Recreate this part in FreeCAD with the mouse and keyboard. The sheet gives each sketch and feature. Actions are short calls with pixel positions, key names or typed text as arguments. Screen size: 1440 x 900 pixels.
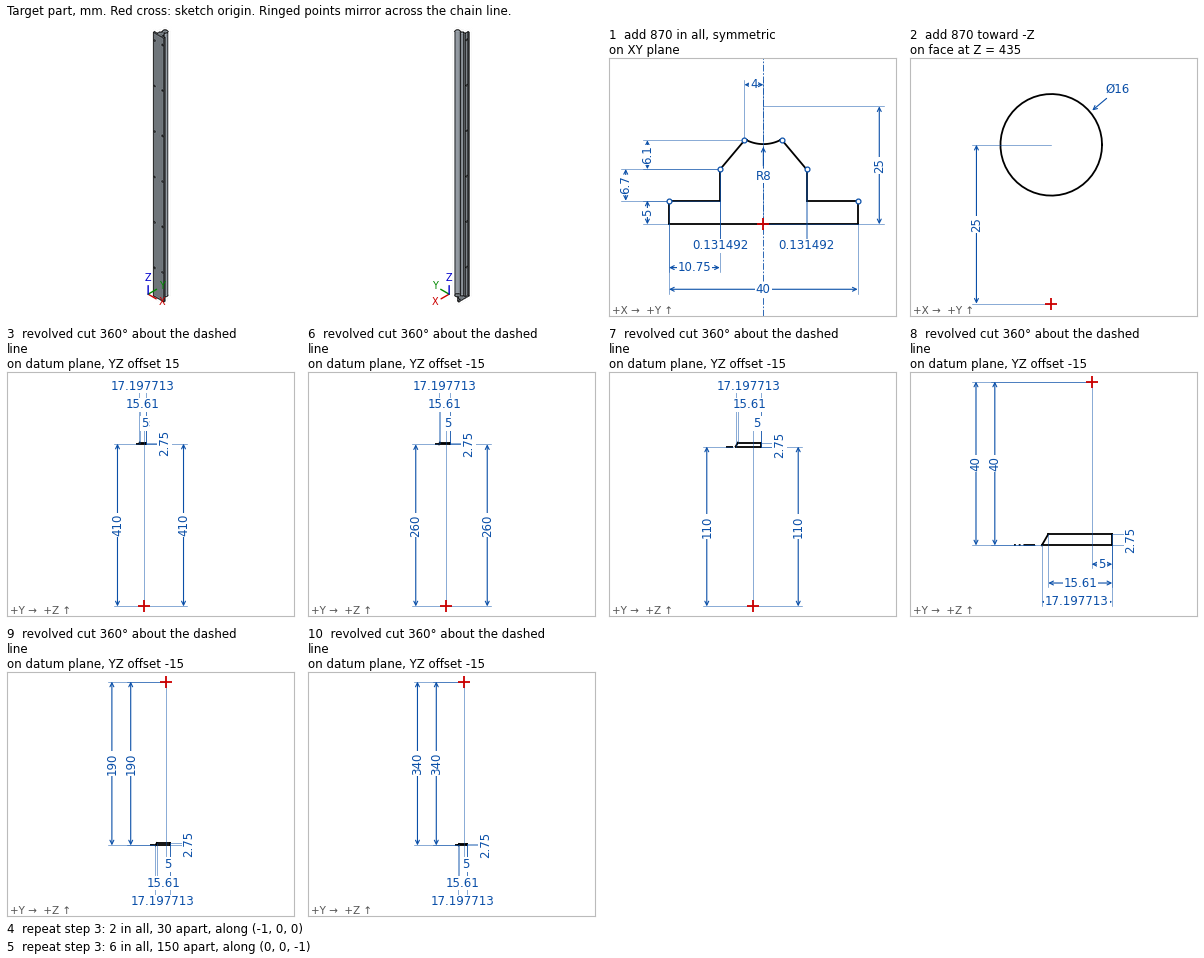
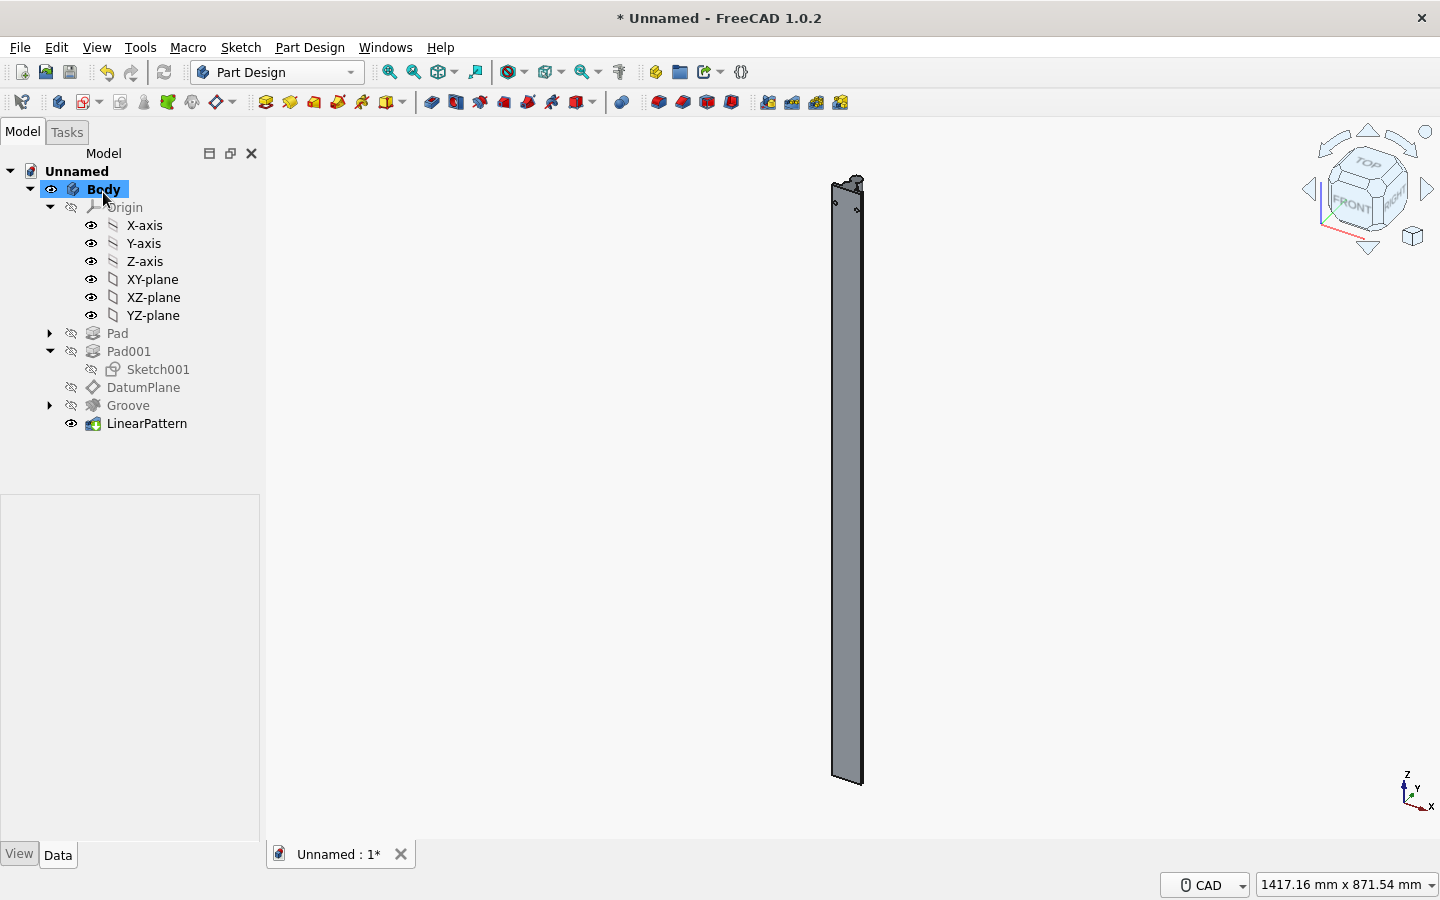
click(116, 405)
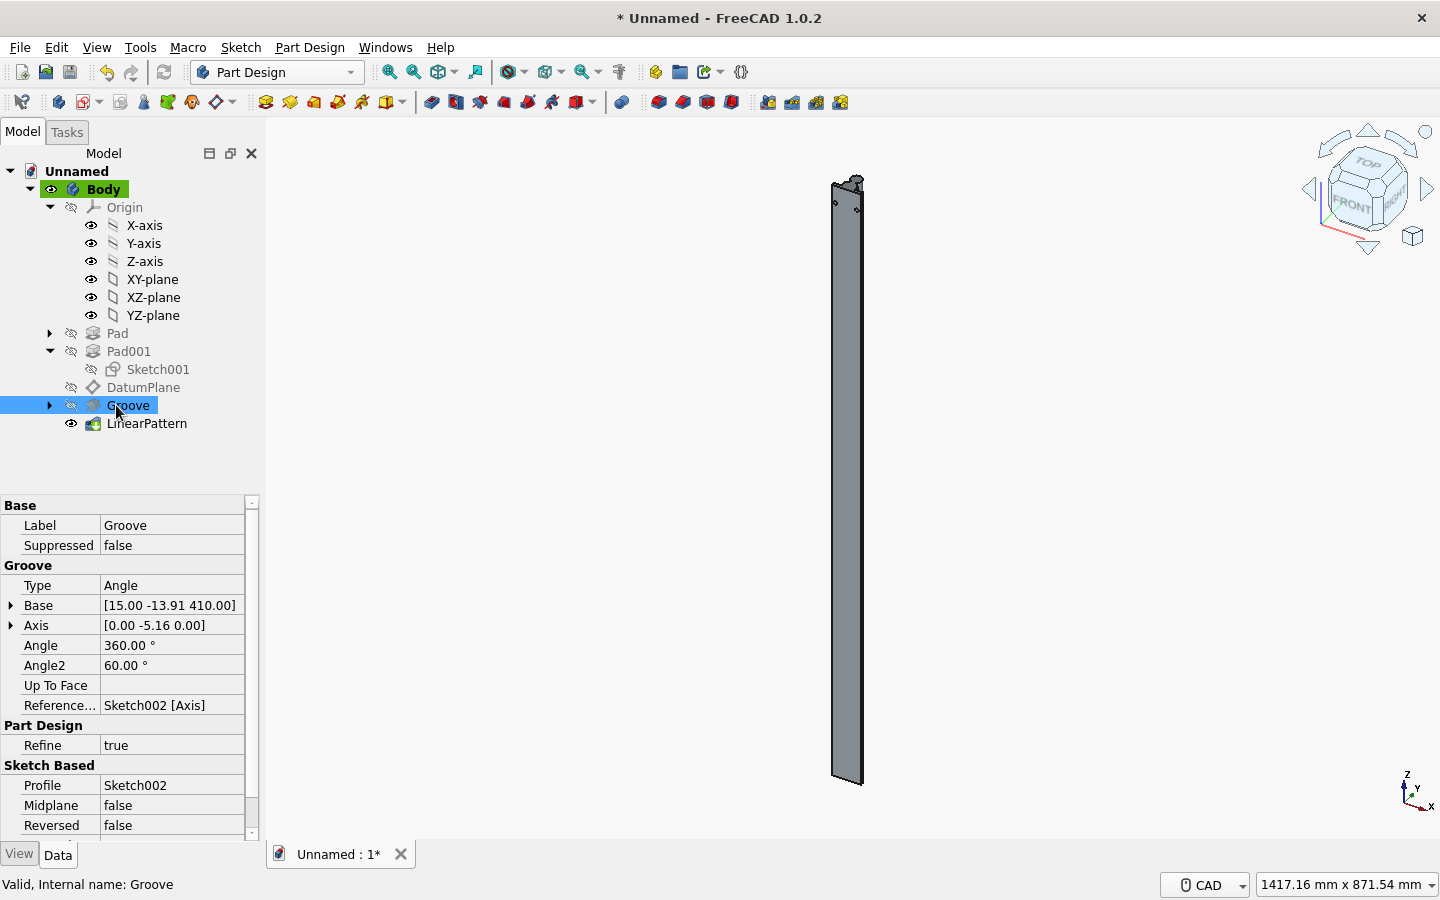
click(792, 102)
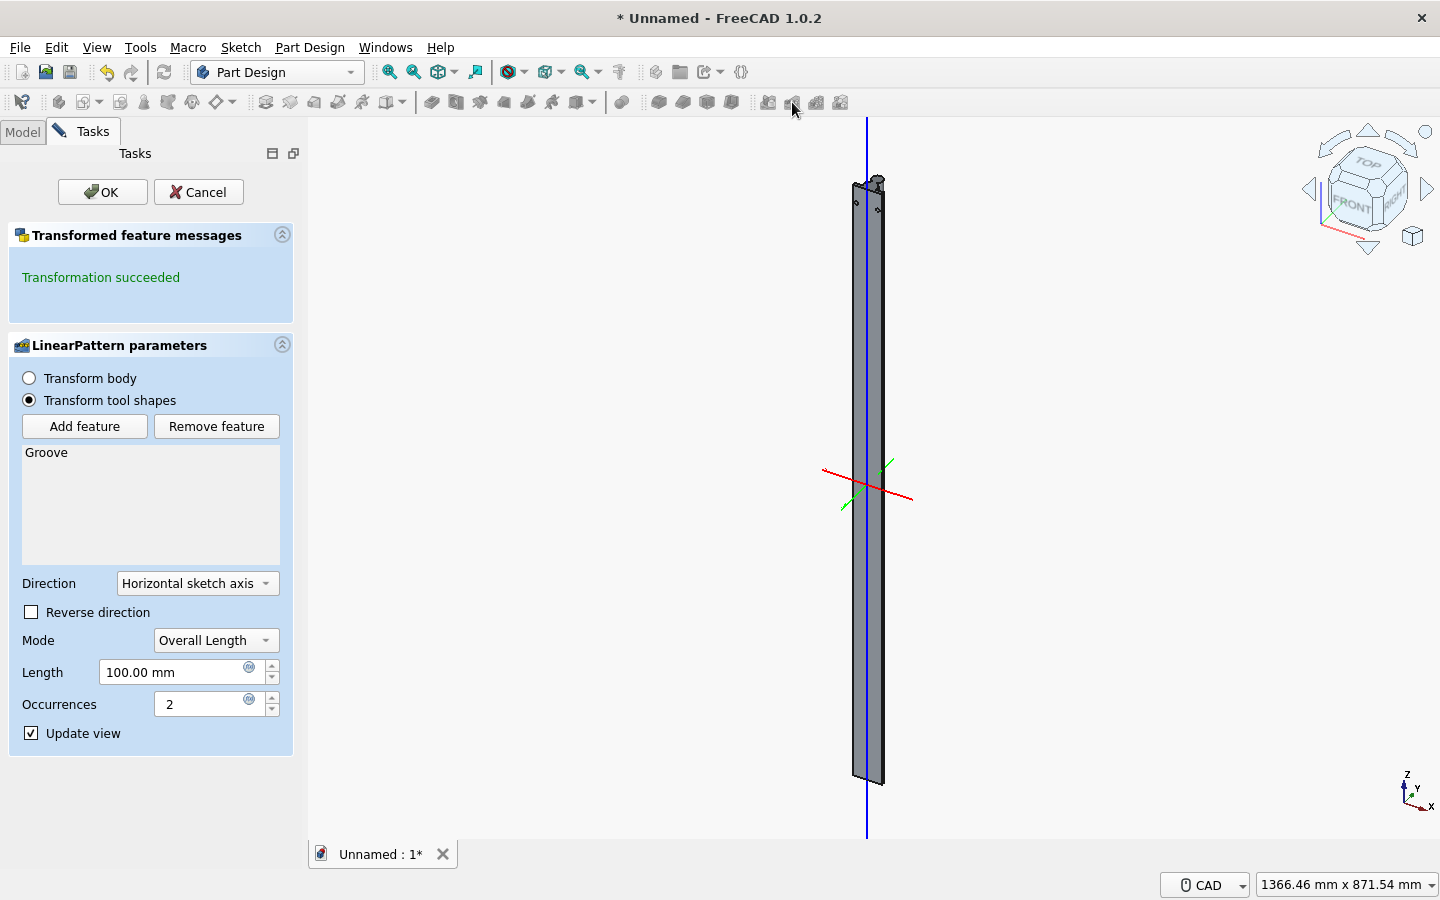
click(198, 584)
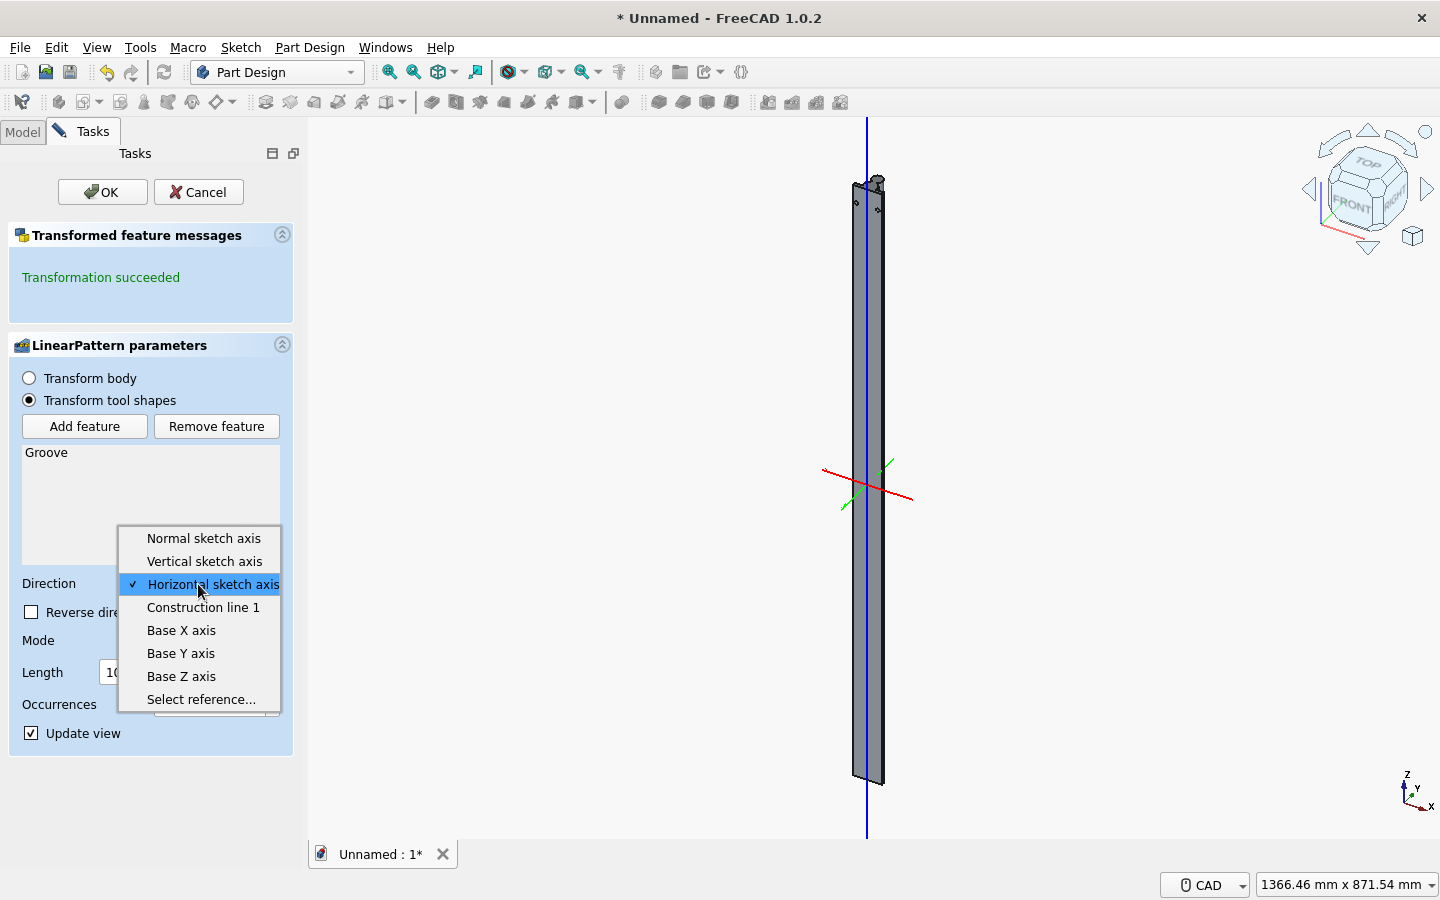
click(198, 676)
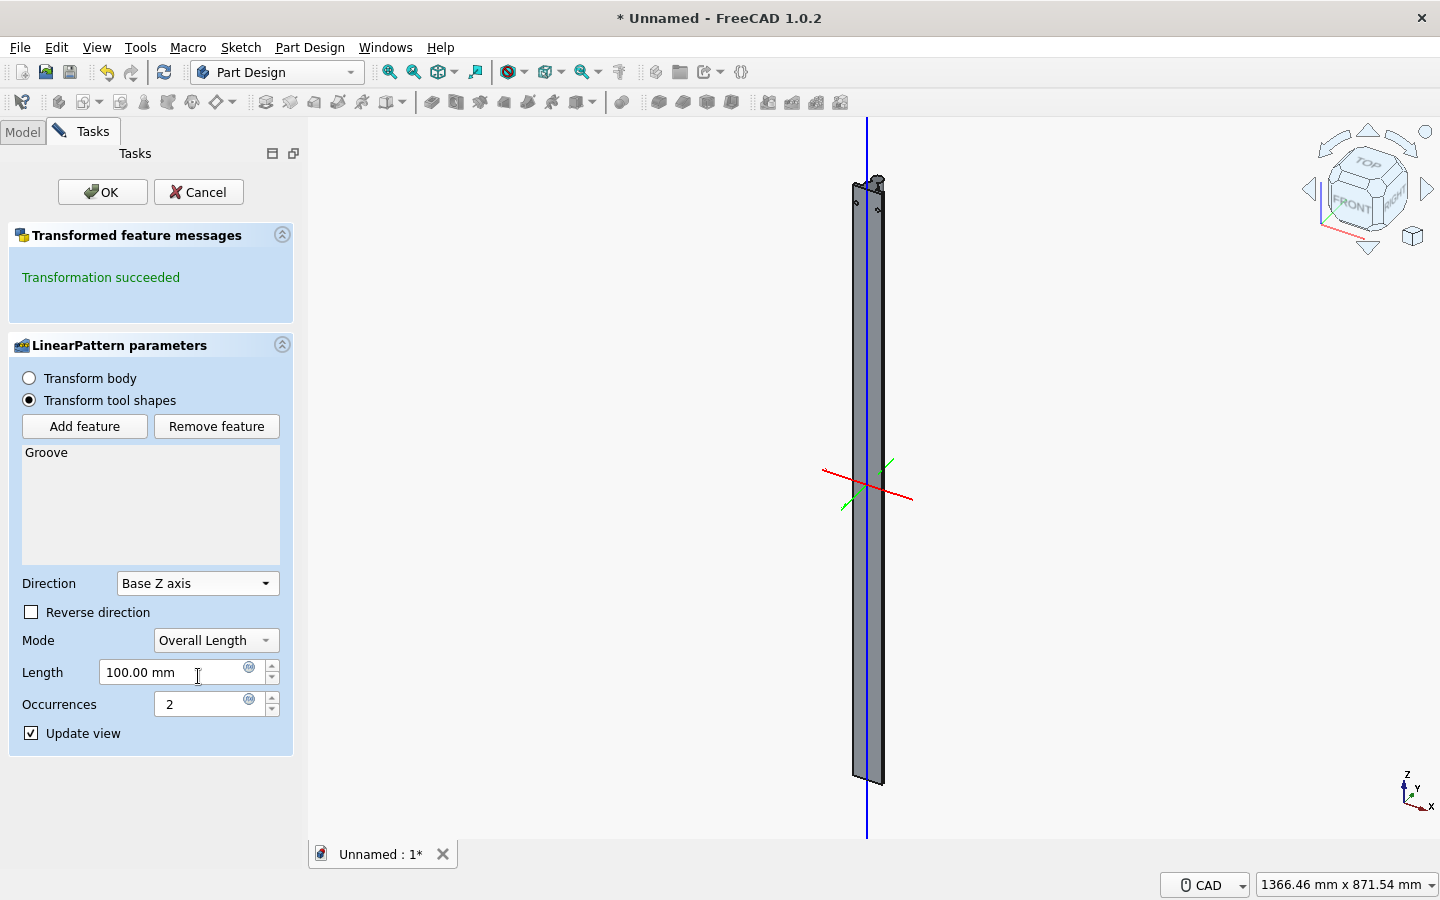
click(217, 640)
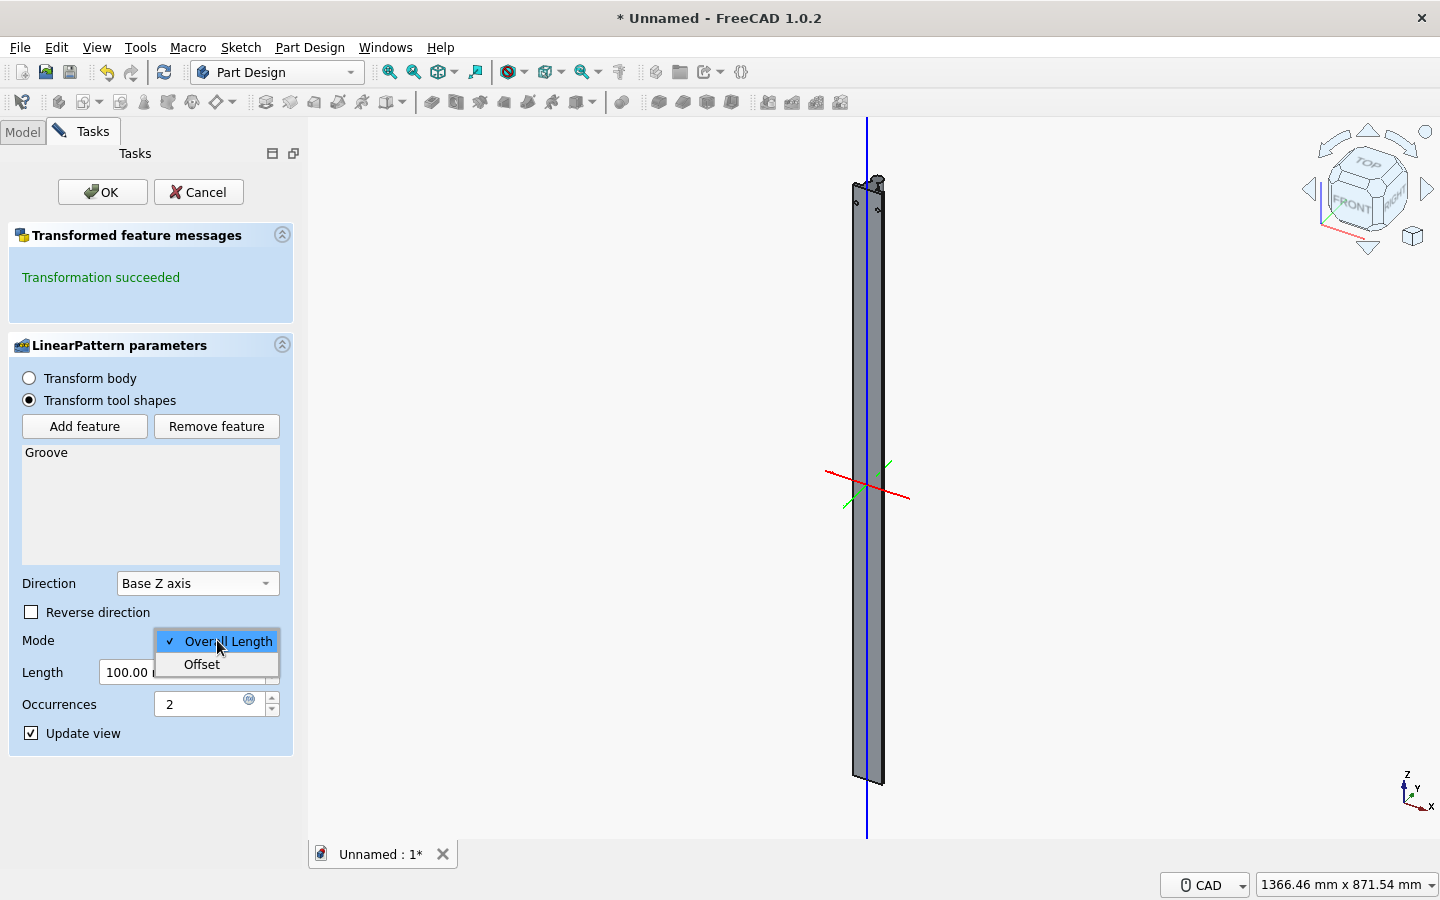
click(216, 664)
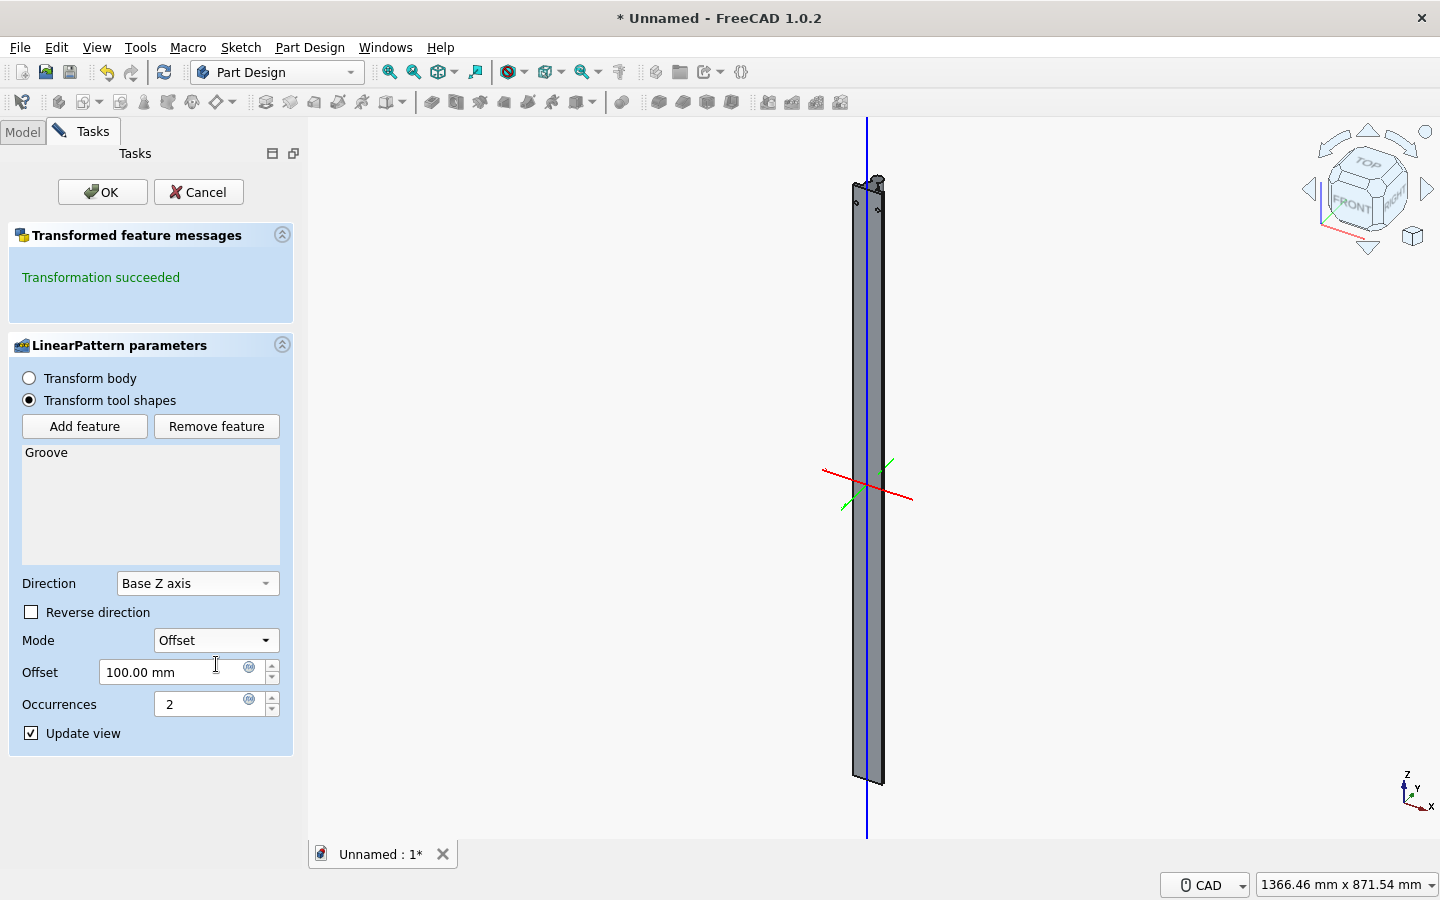
triple_click(182, 672)